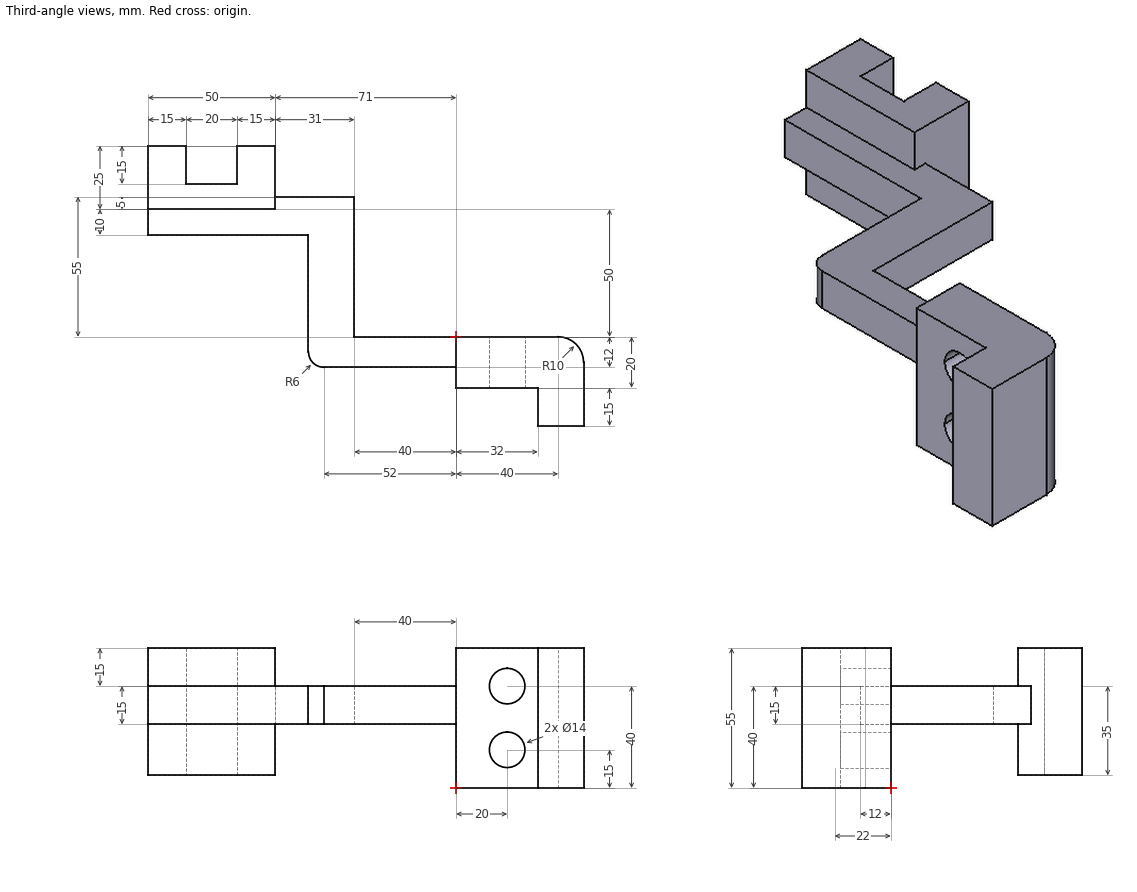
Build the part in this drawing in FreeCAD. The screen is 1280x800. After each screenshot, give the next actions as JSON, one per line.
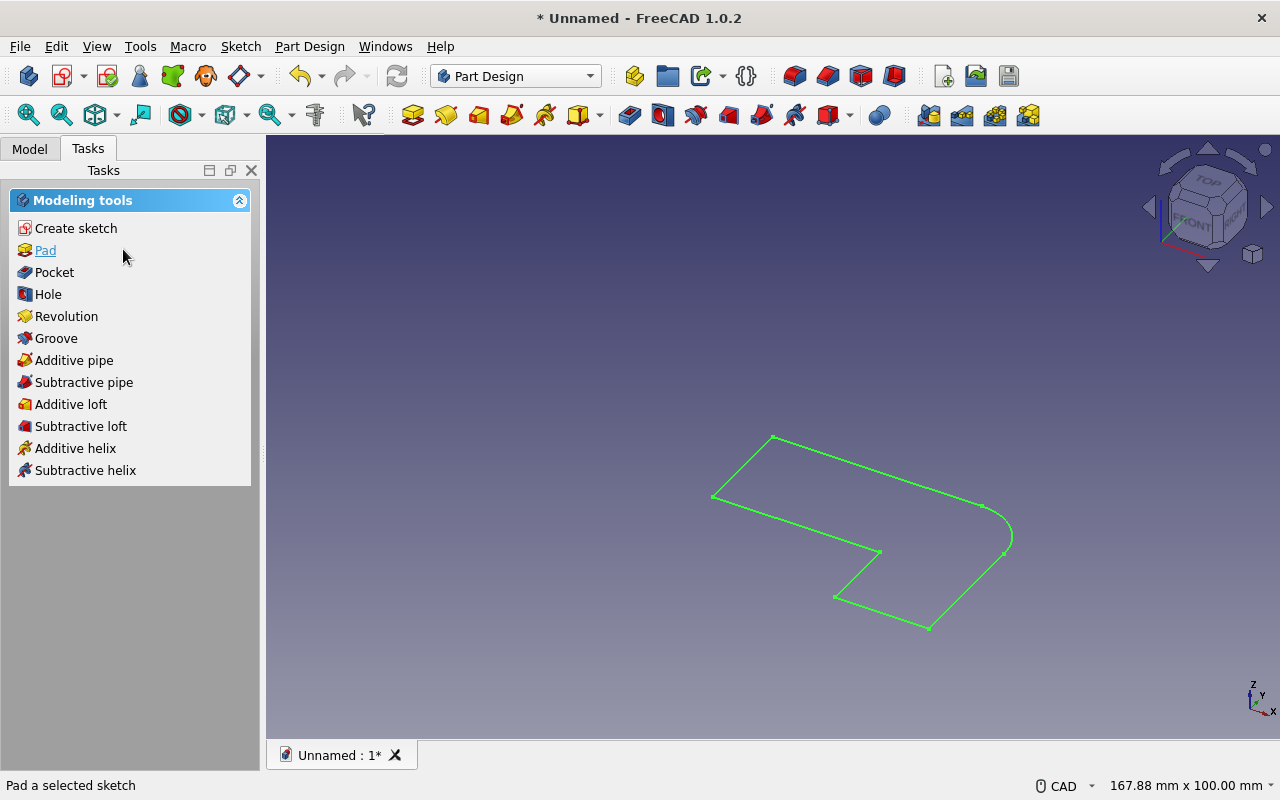
{"action": "left_click", "coordinate": [413, 116]}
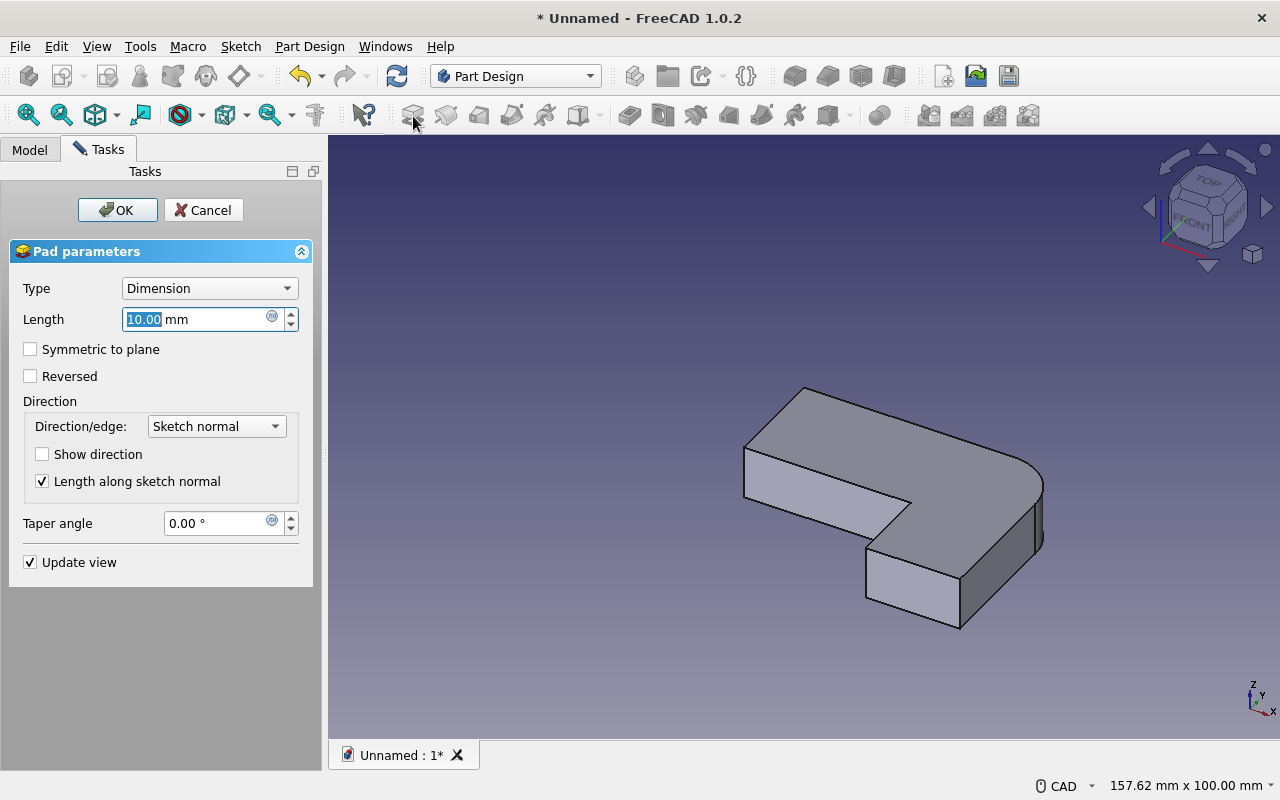
{"action": "type", "text": "55"}
{"action": "key", "text": "Tab"}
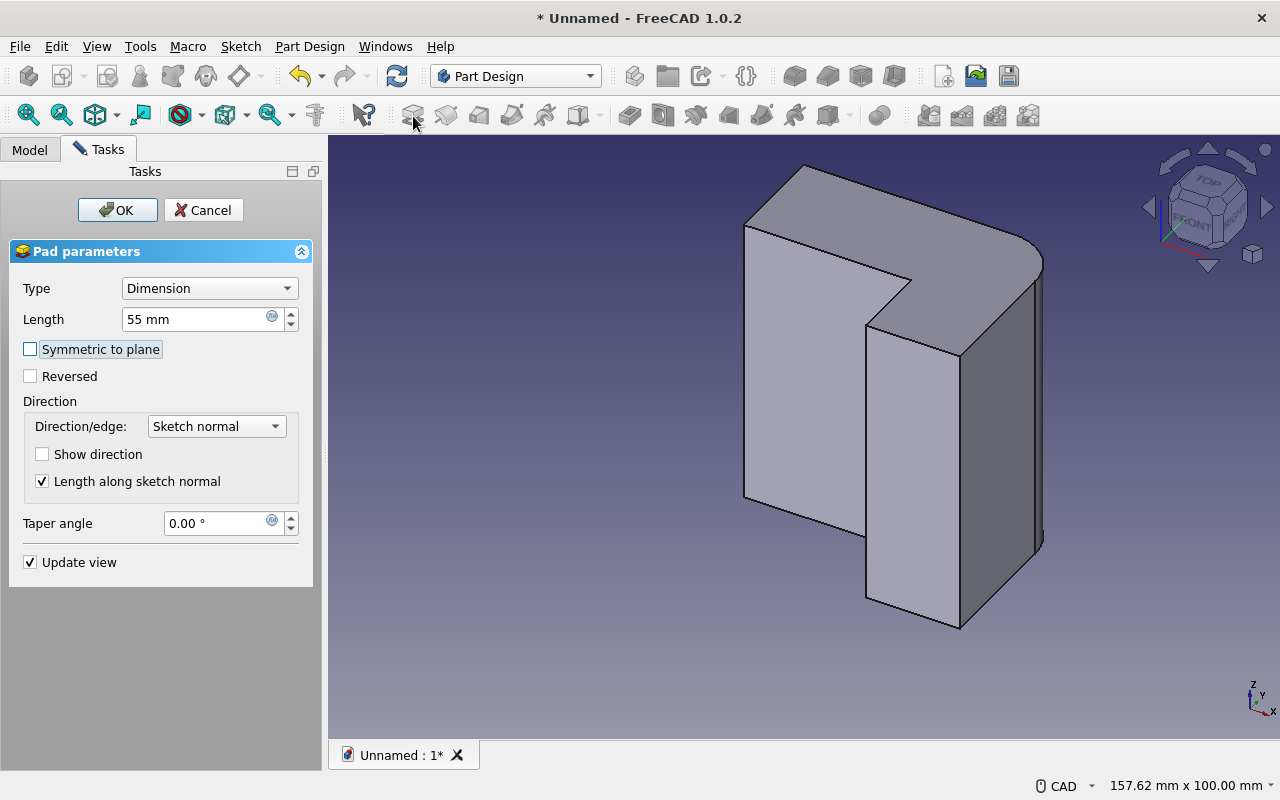
{"action": "left_click", "coordinate": [118, 210]}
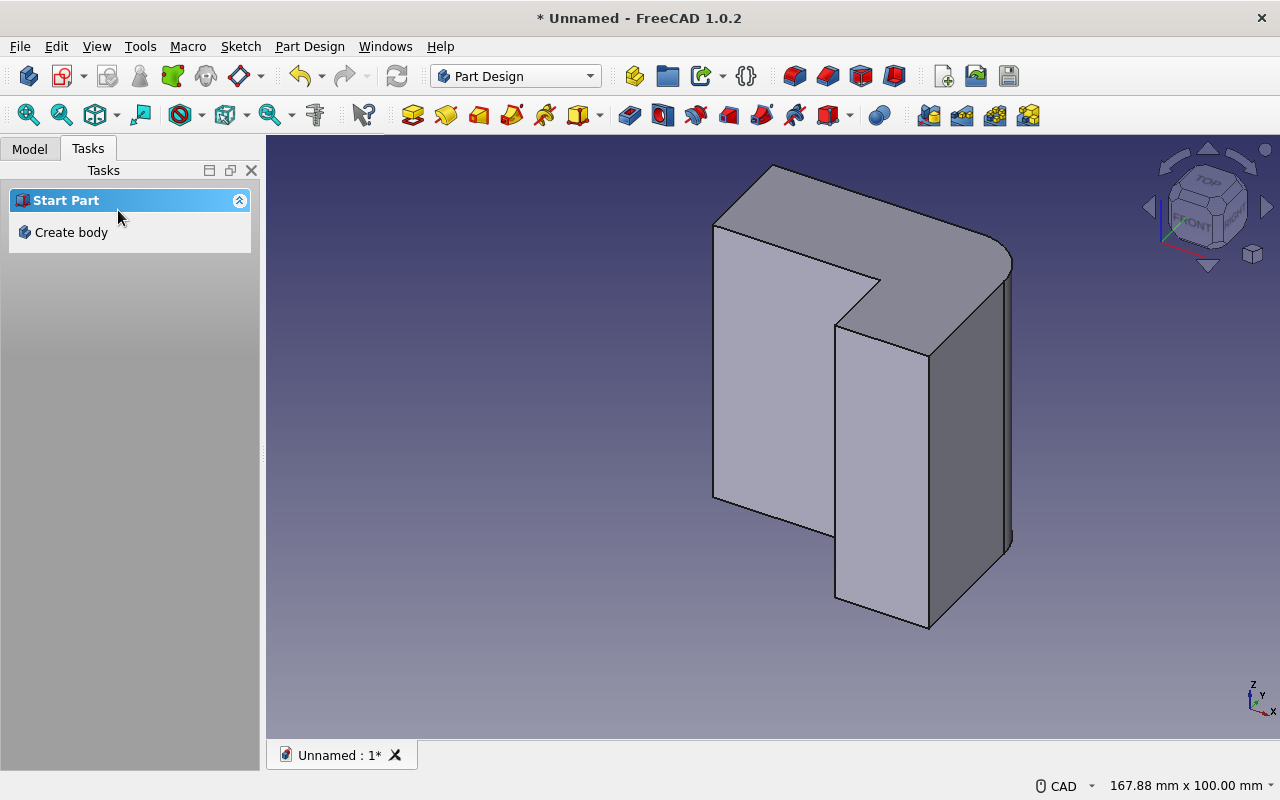
{"action": "key", "text": "4"}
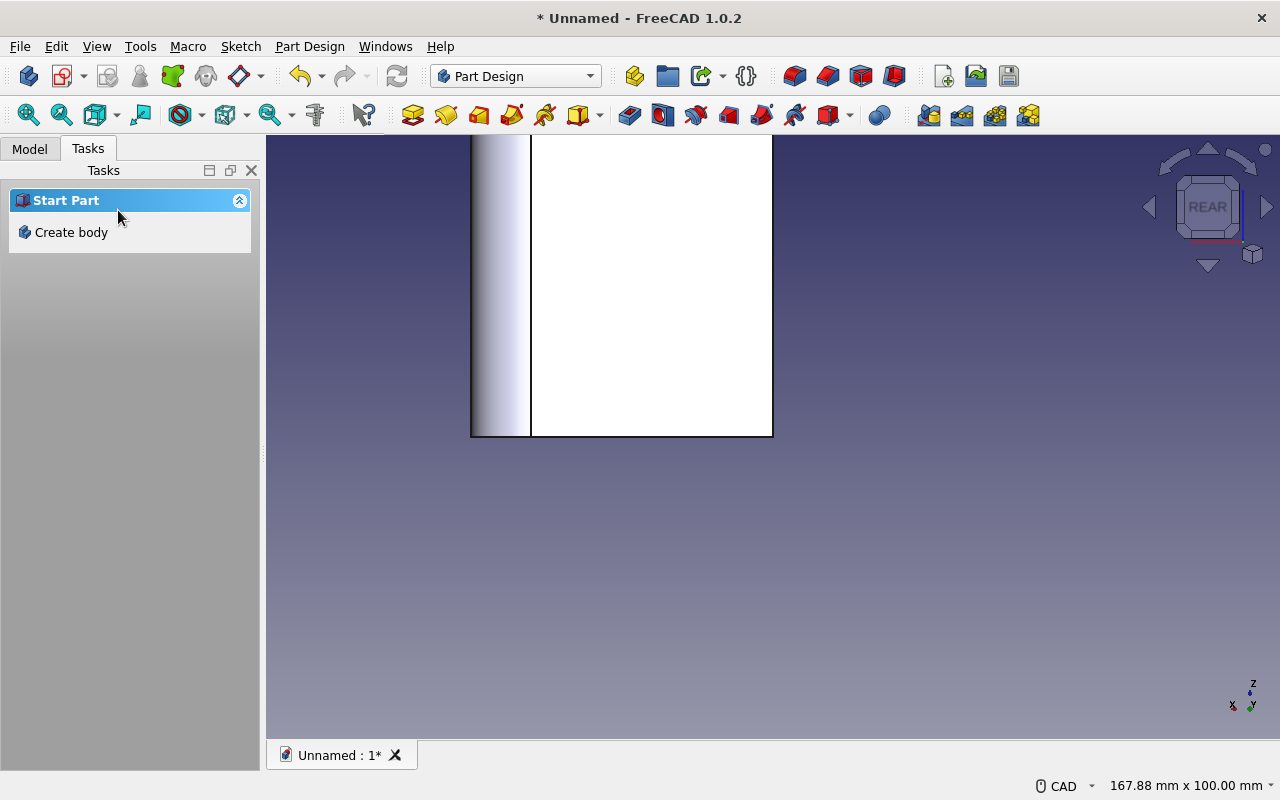
{"action": "left_click", "coordinate": [29, 116]}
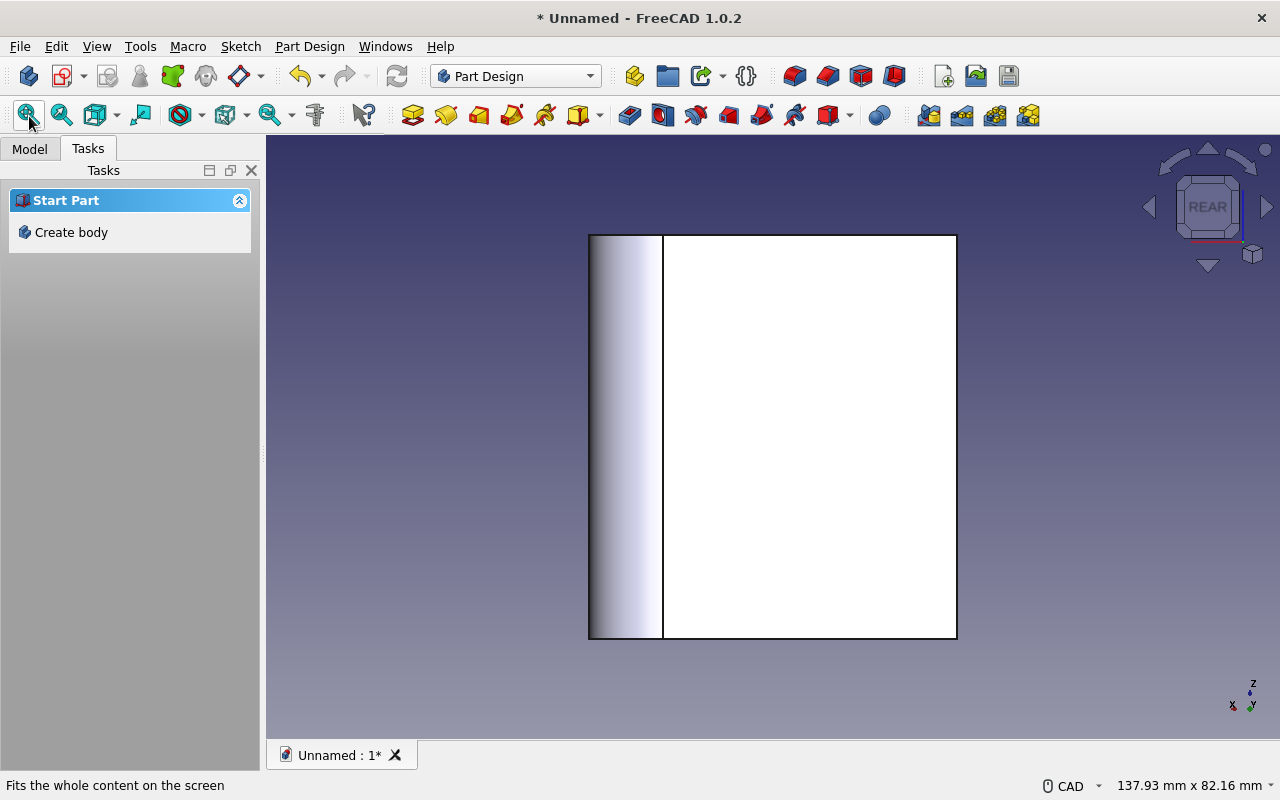
{"action": "left_click", "coordinate": [810, 436]}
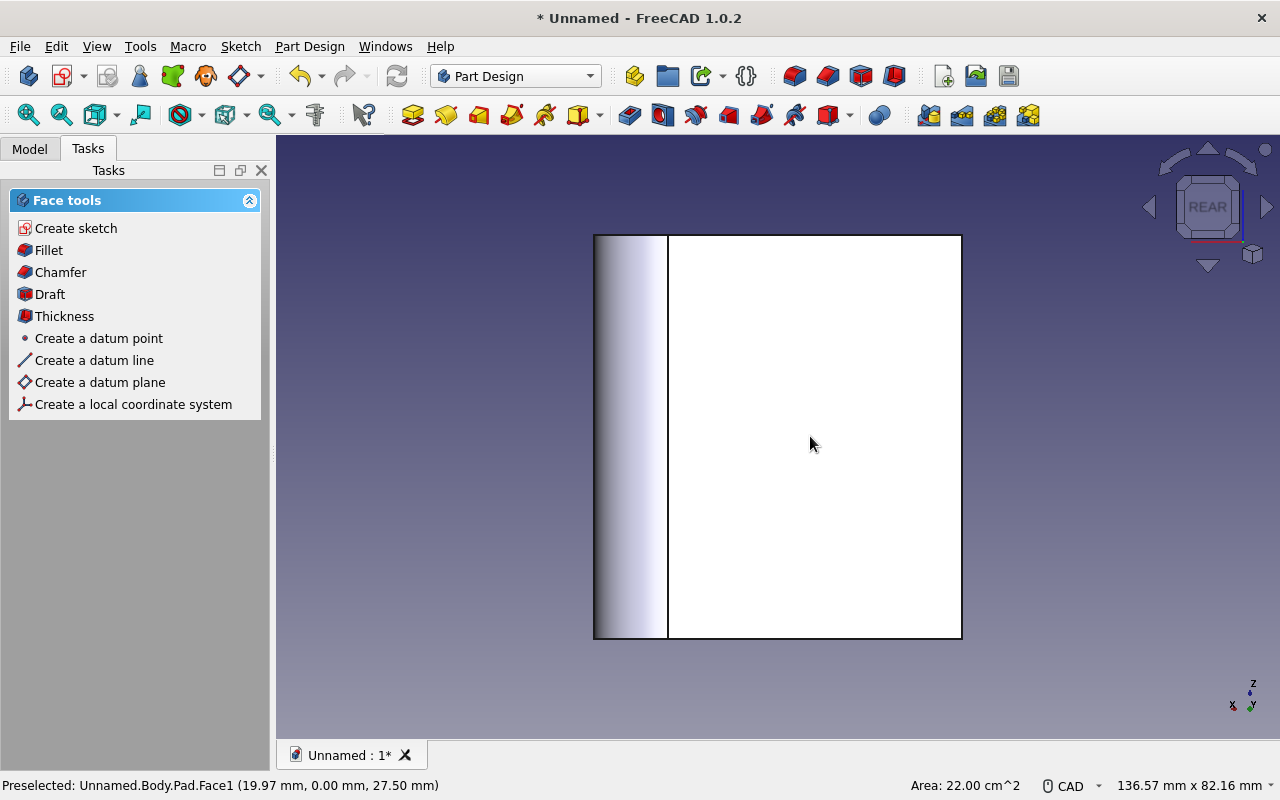
{"action": "left_click", "coordinate": [62, 76]}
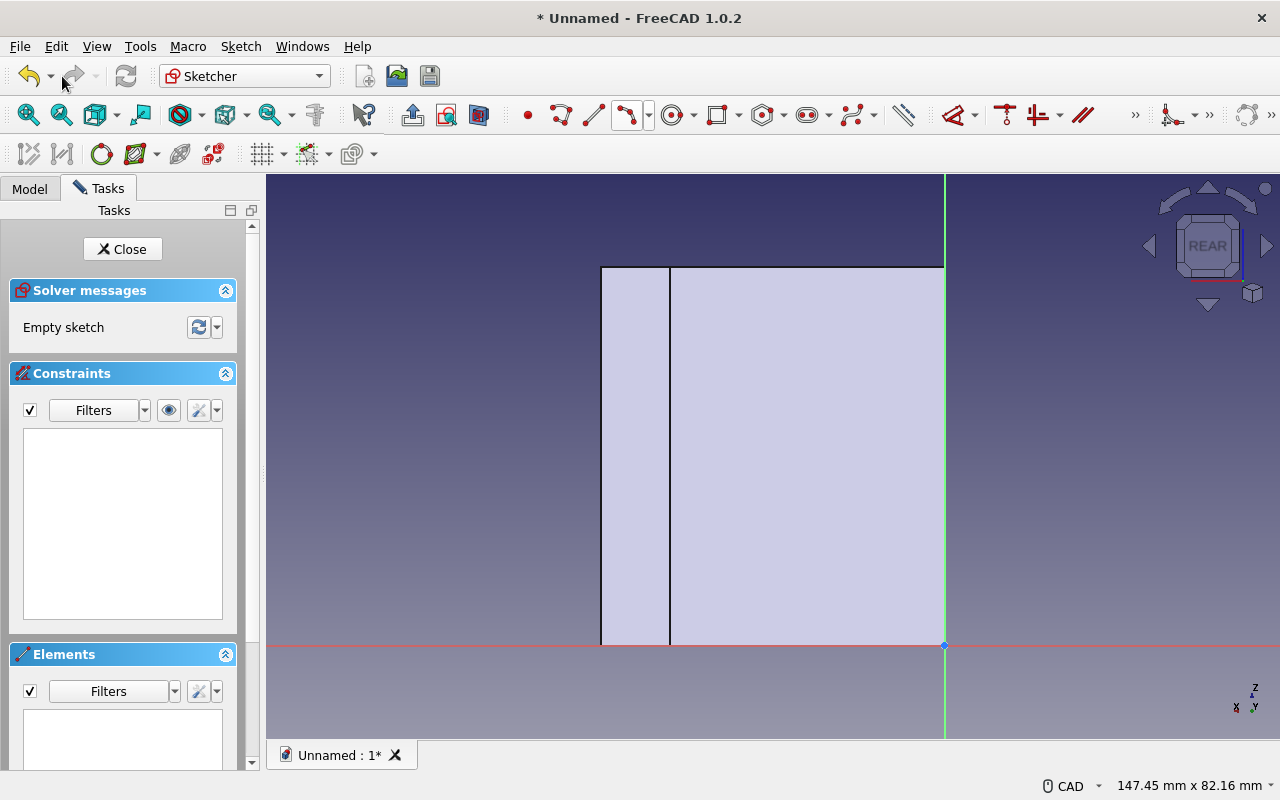
{"action": "left_click", "coordinate": [672, 116]}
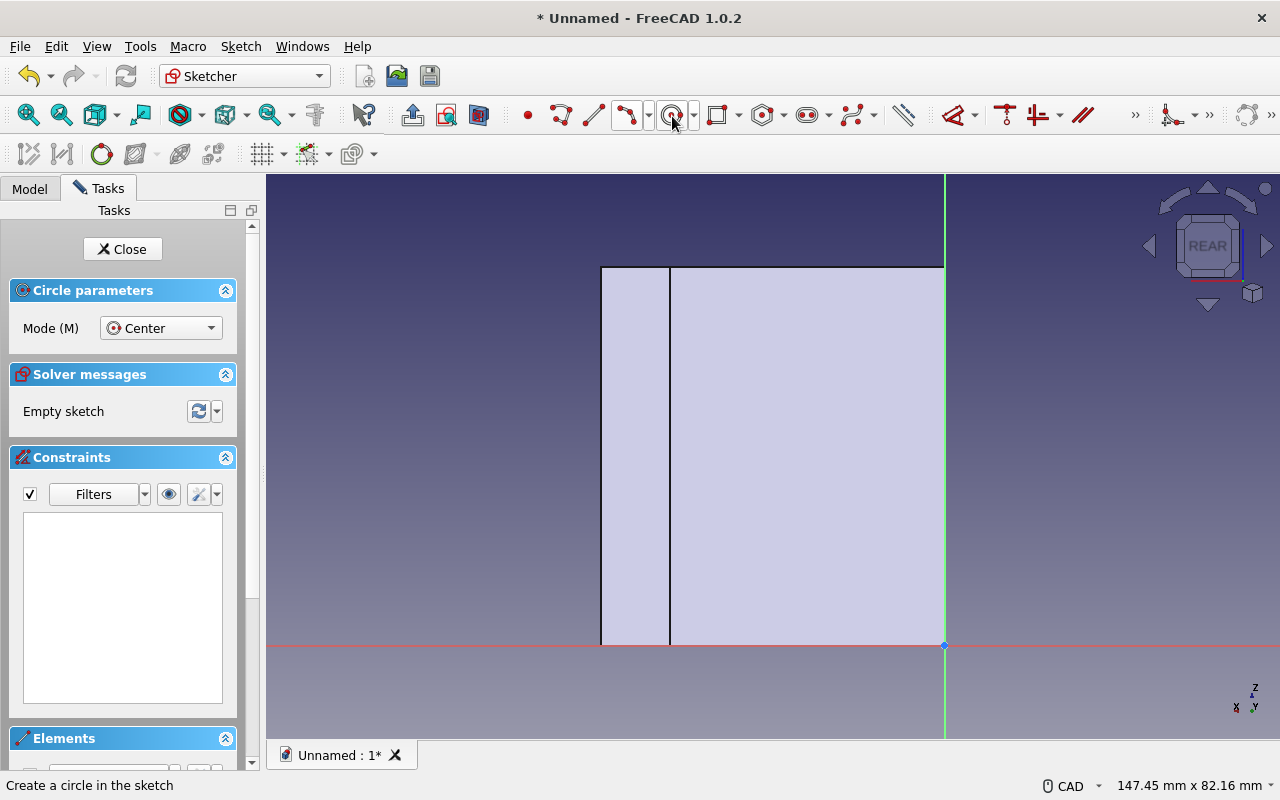
{"action": "left_click", "coordinate": [807, 542]}
{"action": "left_click", "coordinate": [841, 508]}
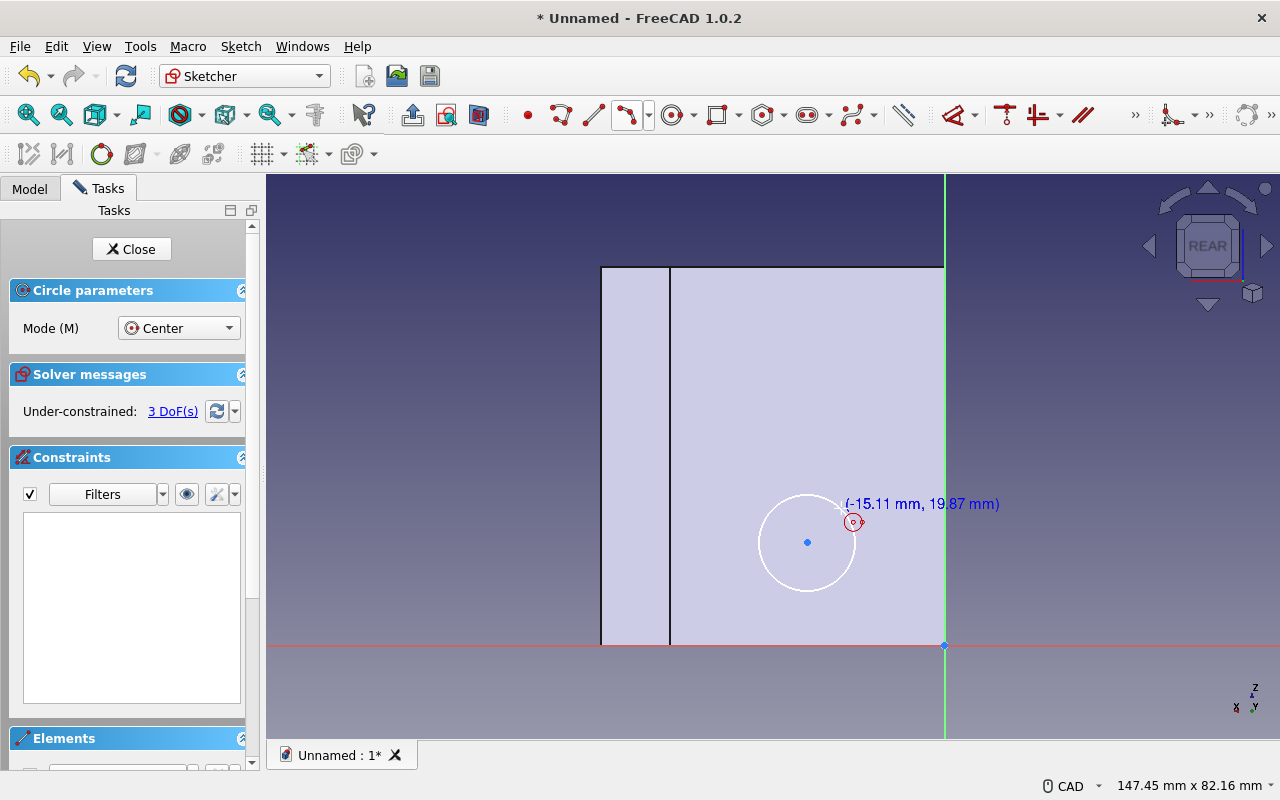
{"action": "left_click", "coordinate": [807, 371]}
{"action": "left_click", "coordinate": [841, 336]}
{"action": "key", "text": "Escape"}